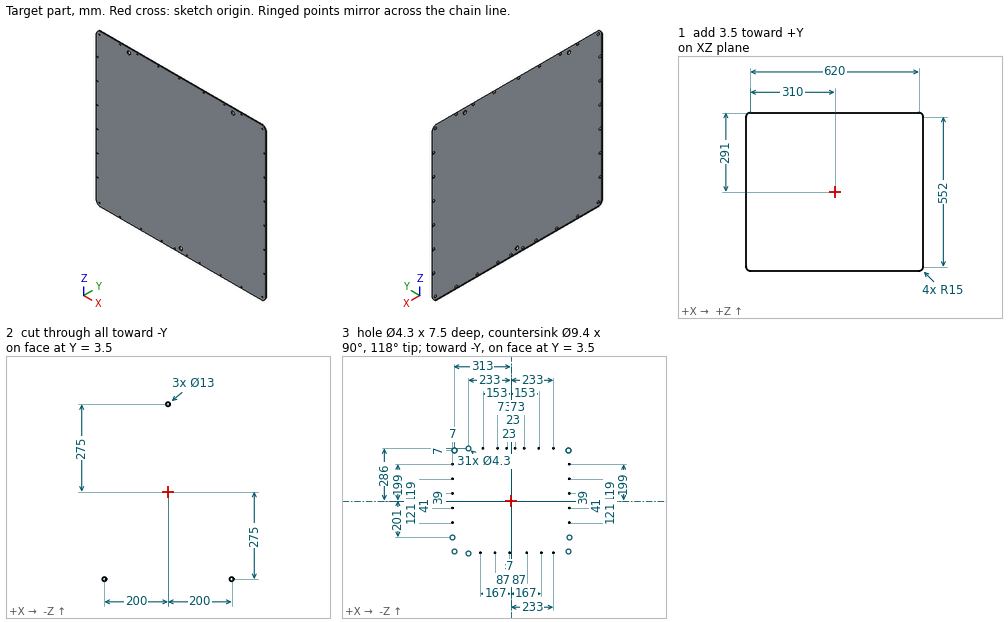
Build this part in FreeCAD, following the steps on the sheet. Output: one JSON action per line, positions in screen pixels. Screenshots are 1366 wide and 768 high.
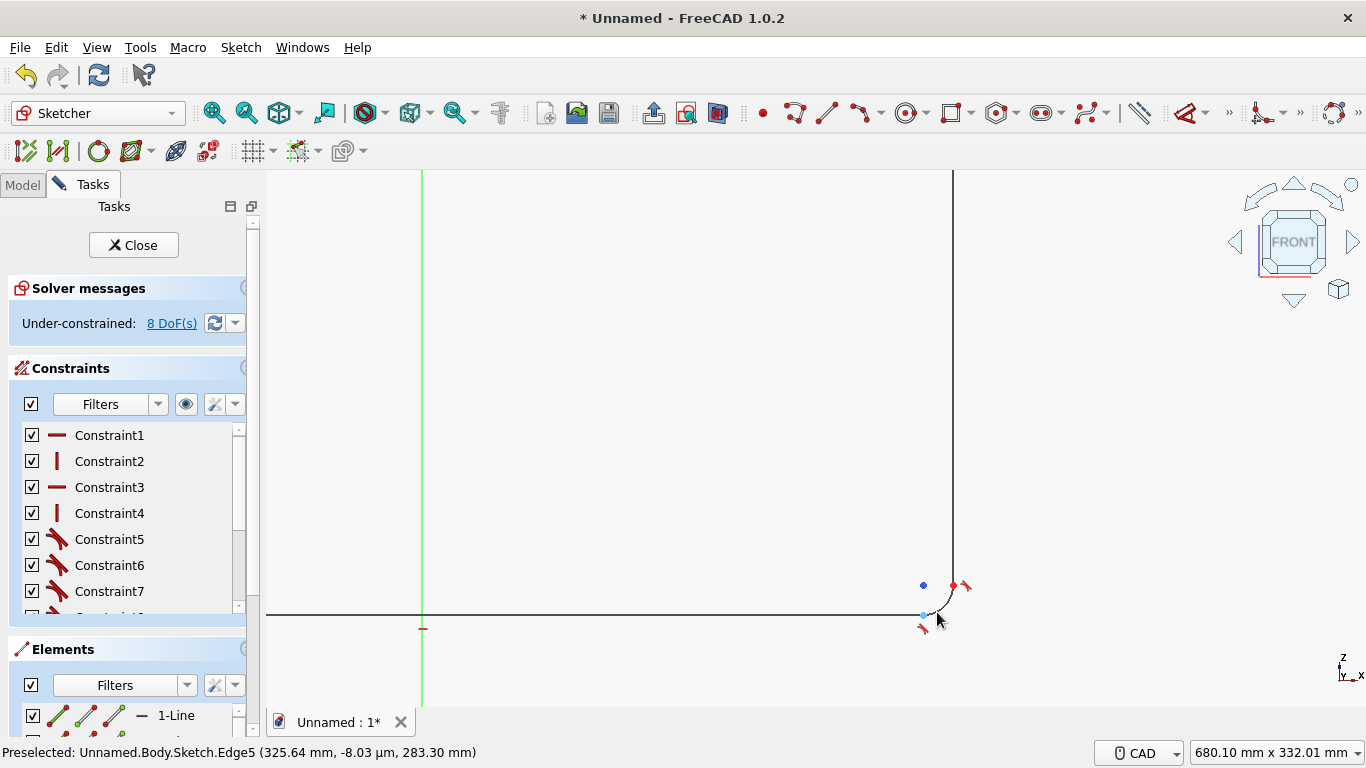
{"action": "left_click", "coordinate": [937, 612]}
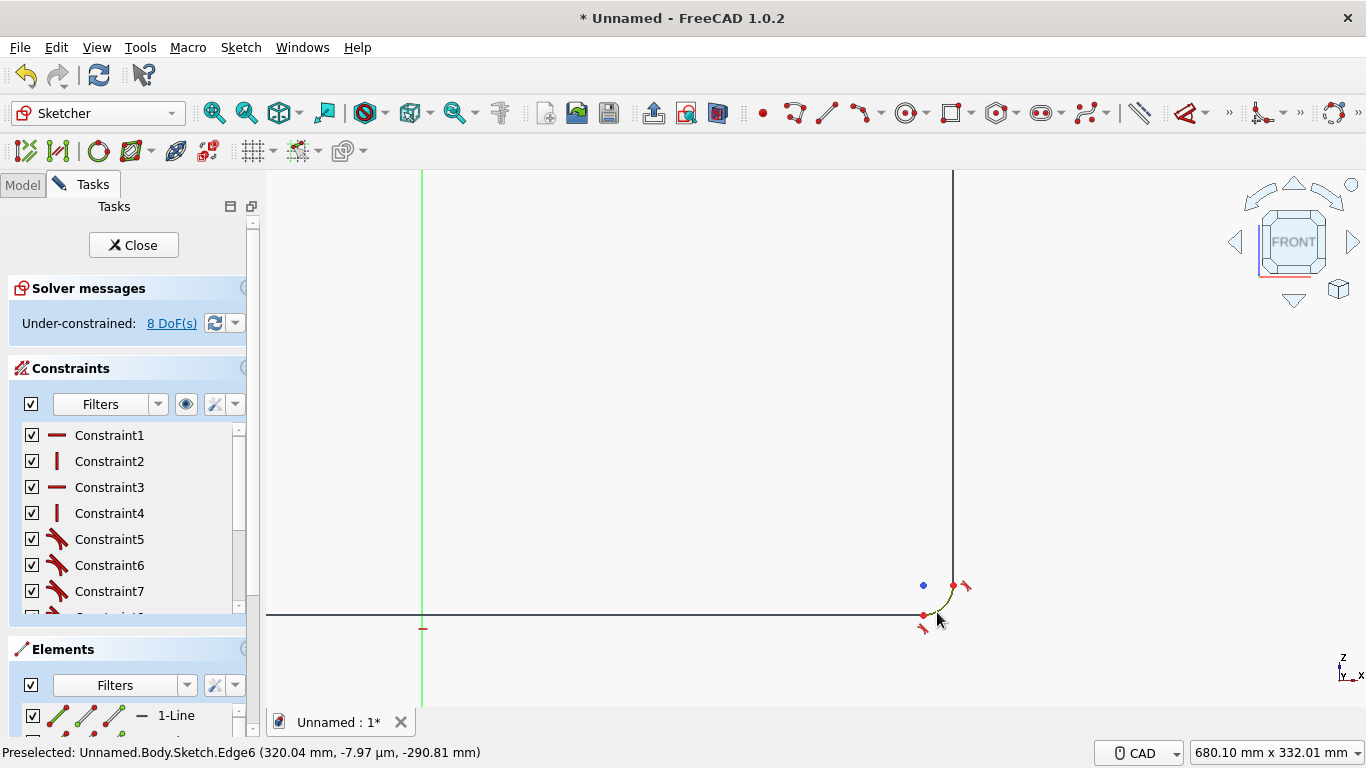
{"action": "scroll", "coordinate": [937, 613], "scroll_direction": "down", "scroll_amount": 5}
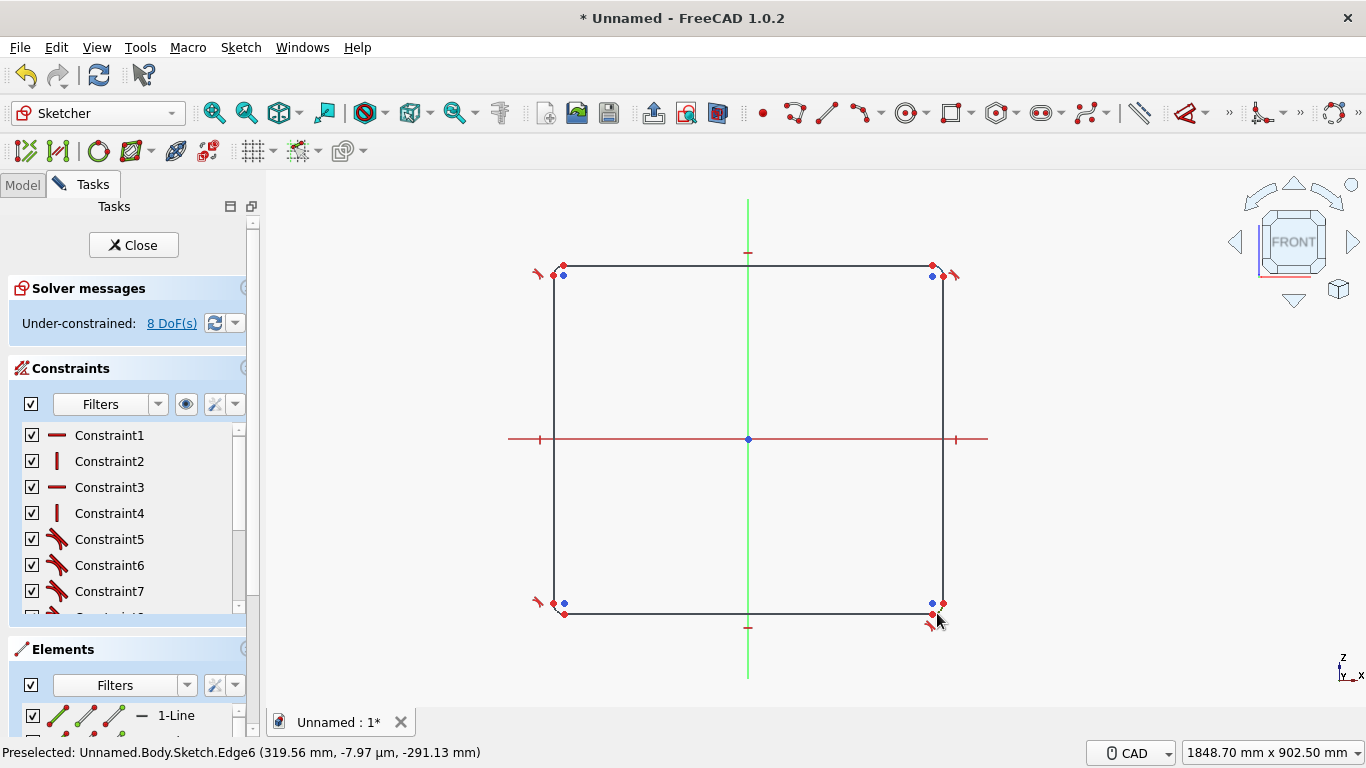
{"action": "scroll", "coordinate": [555, 608], "scroll_direction": "up", "scroll_amount": 6}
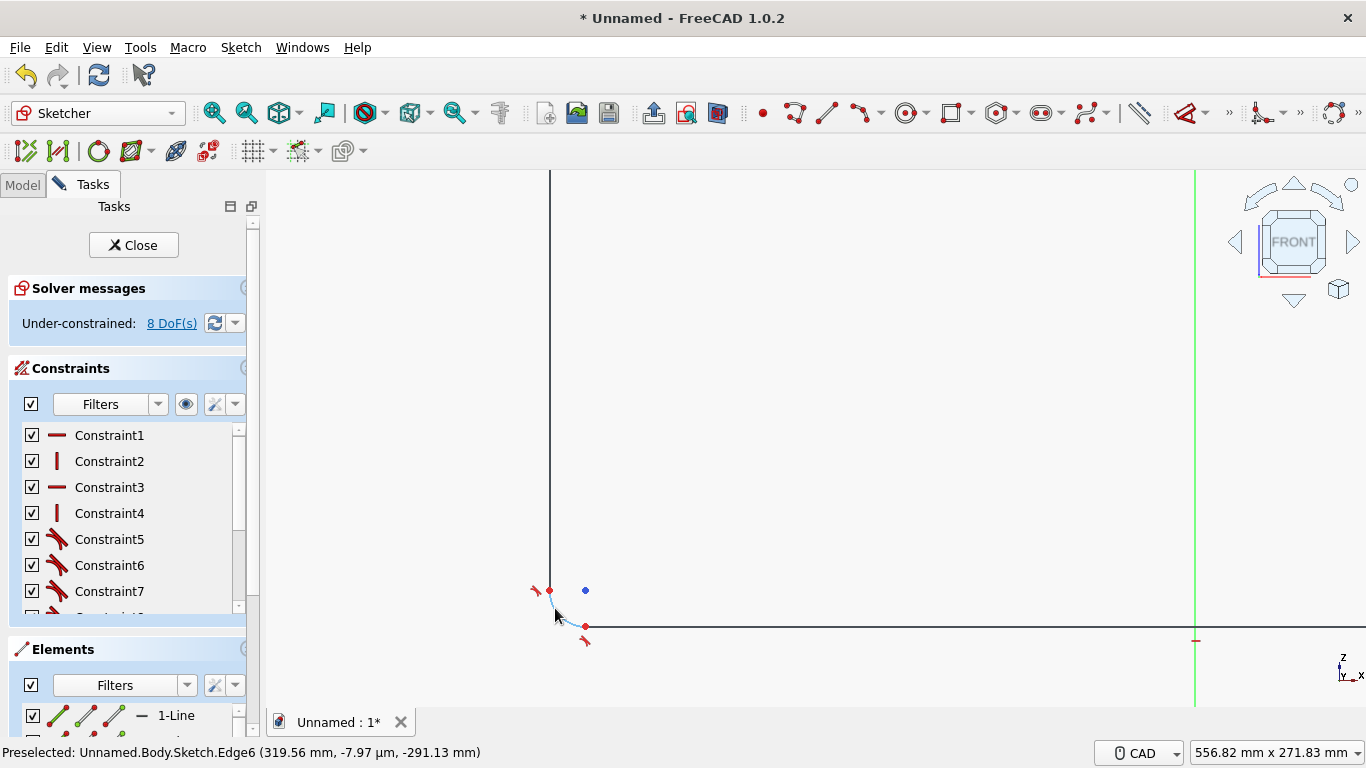
{"action": "left_click", "coordinate": [554, 607]}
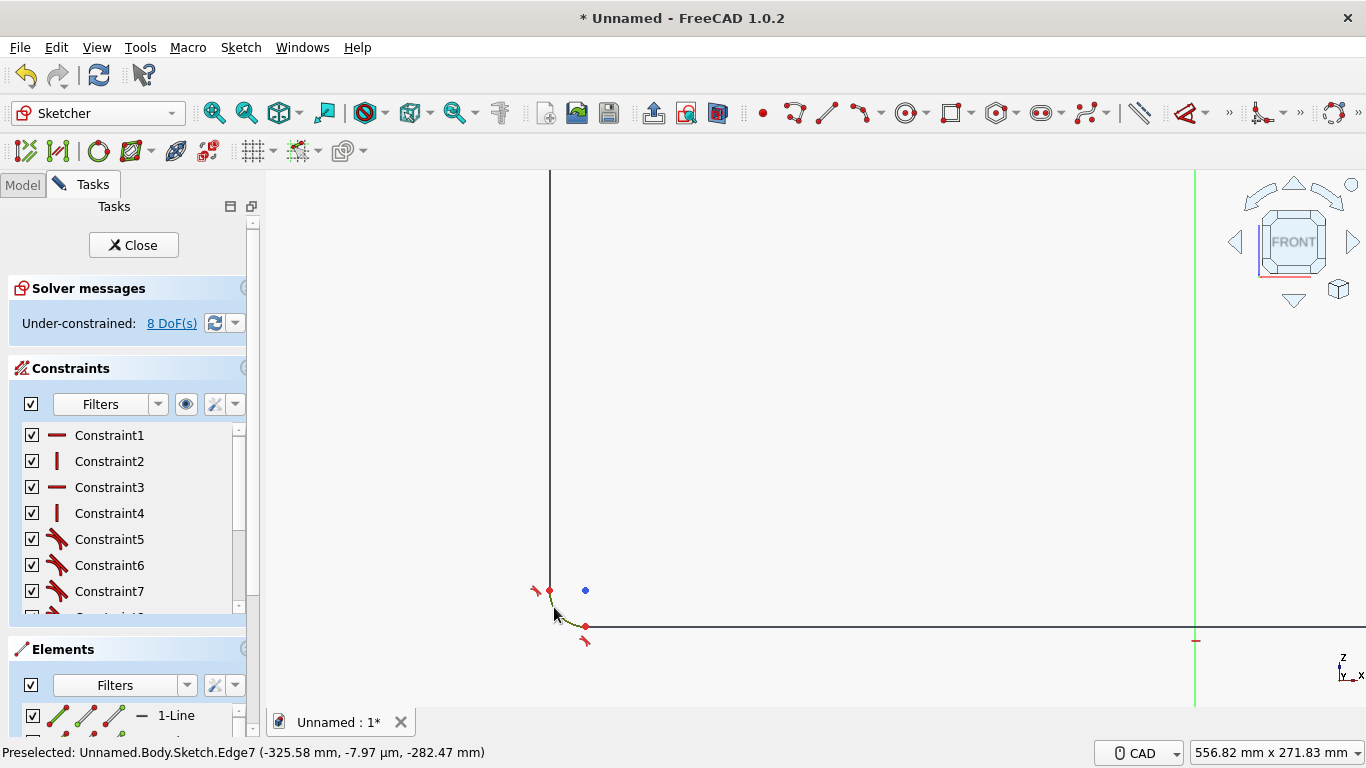
{"action": "scroll", "coordinate": [554, 608], "scroll_direction": "down", "scroll_amount": 6}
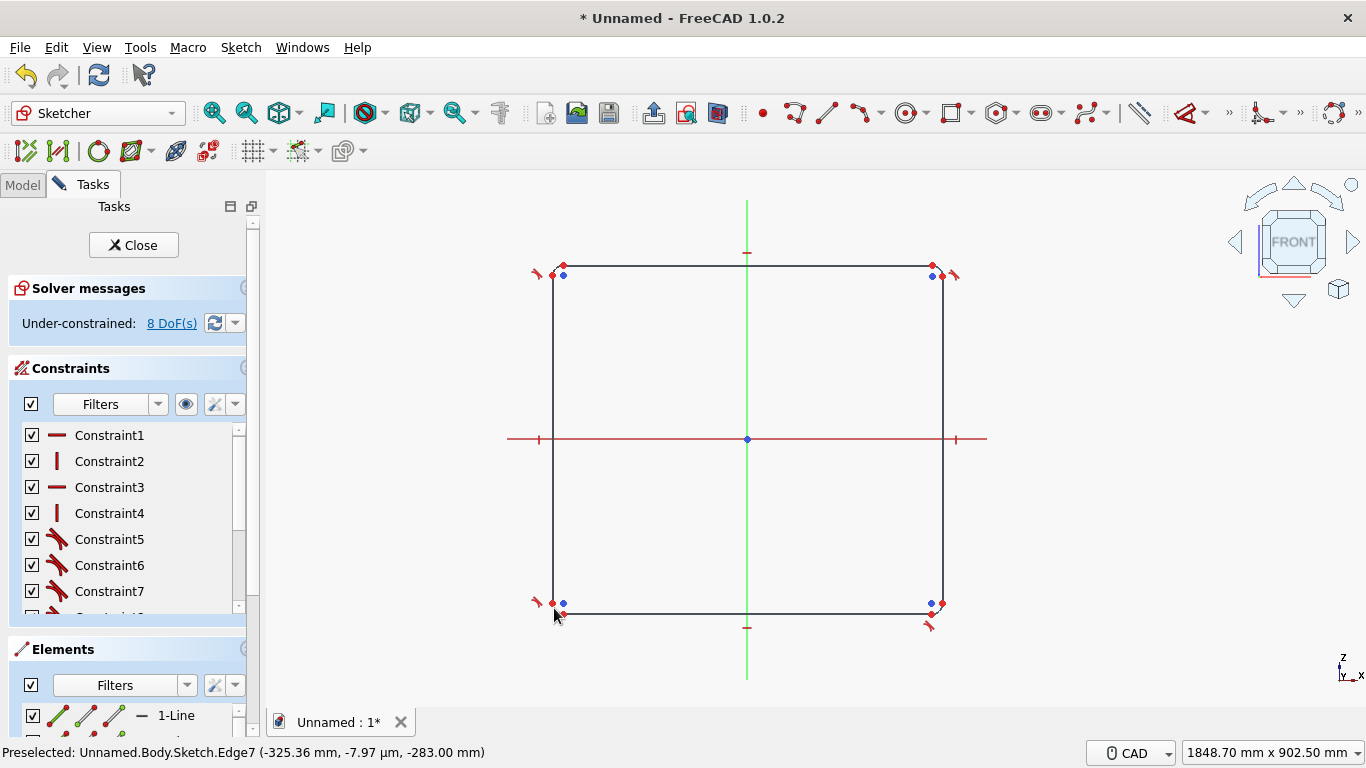
{"action": "scroll", "coordinate": [559, 267], "scroll_direction": "up", "scroll_amount": 6}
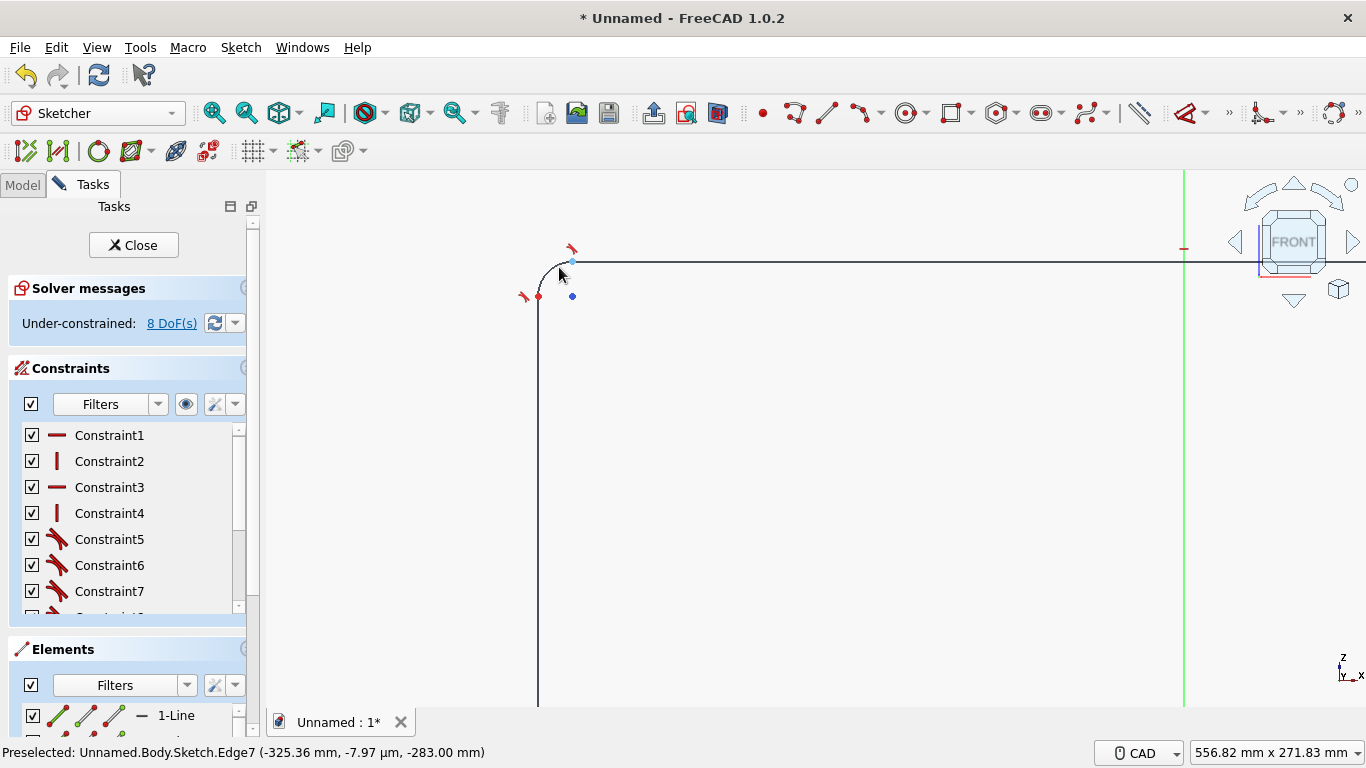
{"action": "left_click", "coordinate": [557, 266]}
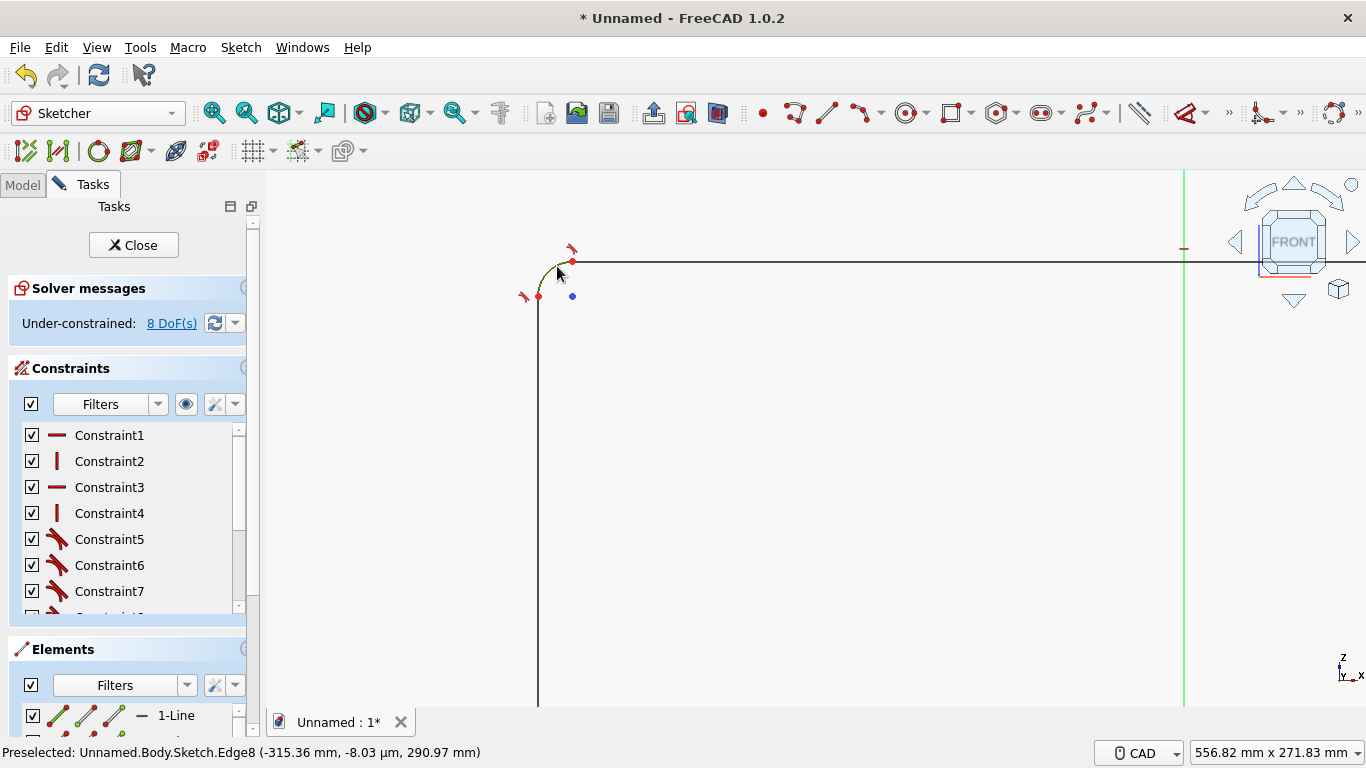
{"action": "key", "text": "e"}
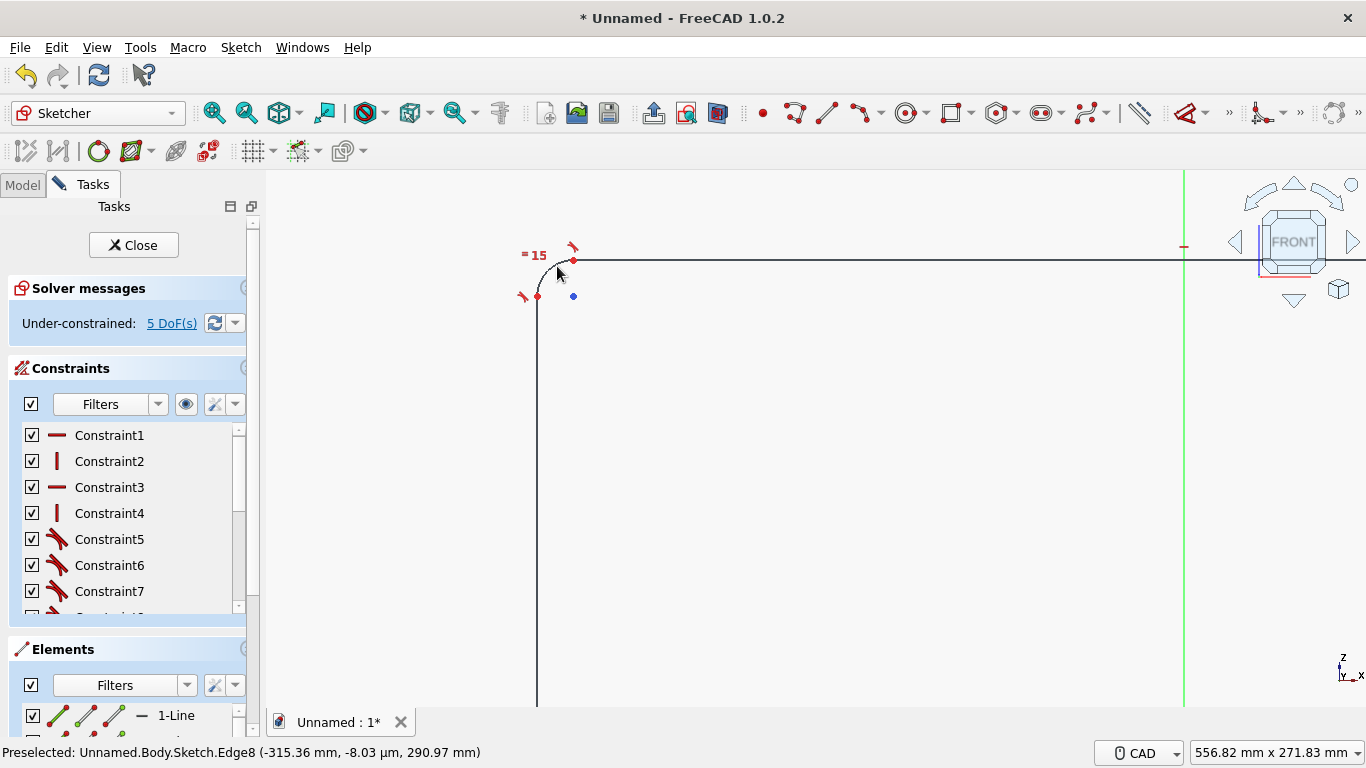
{"action": "left_click", "coordinate": [1186, 114]}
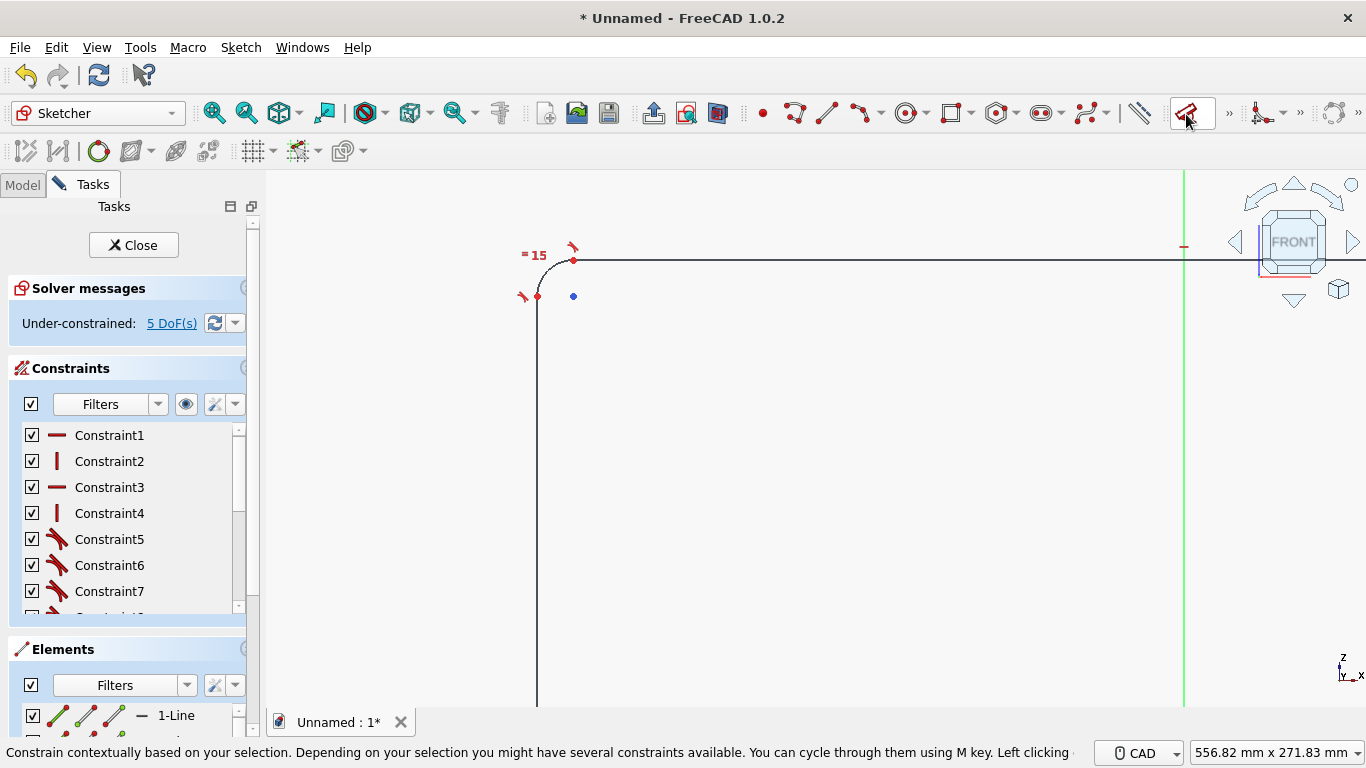
{"action": "scroll", "coordinate": [559, 266], "scroll_direction": "down", "scroll_amount": 6}